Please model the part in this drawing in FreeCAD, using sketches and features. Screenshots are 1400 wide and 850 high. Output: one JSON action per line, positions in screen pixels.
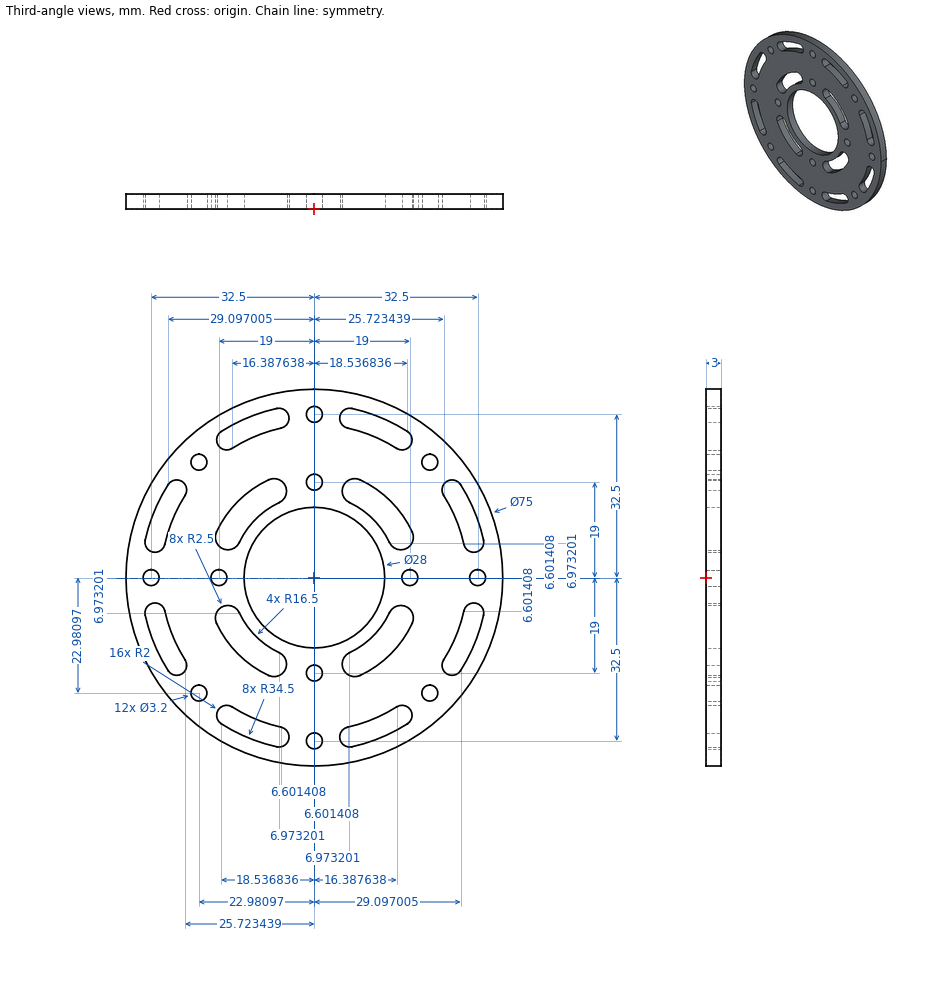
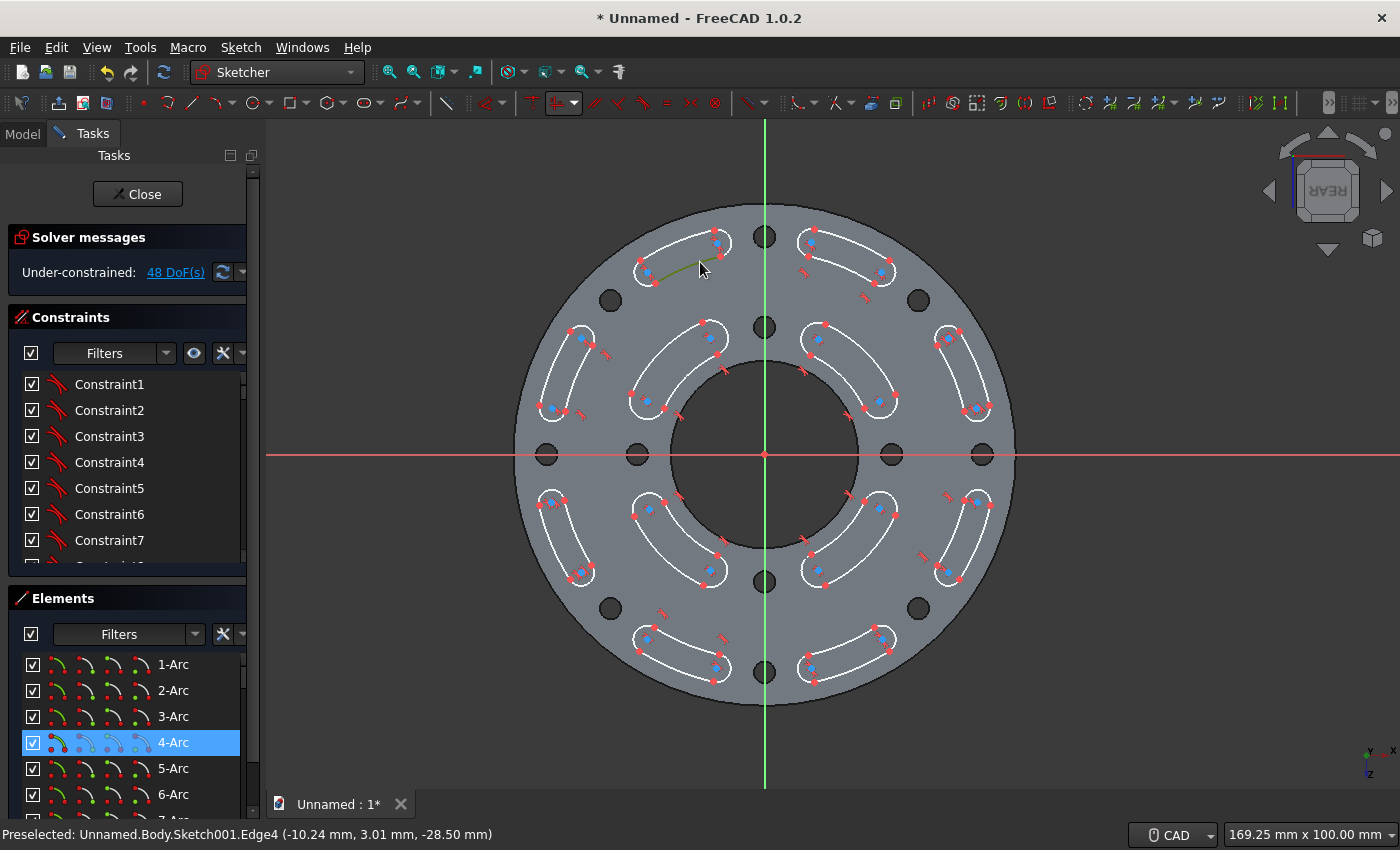
{"action": "left_click", "coordinate": [856, 273]}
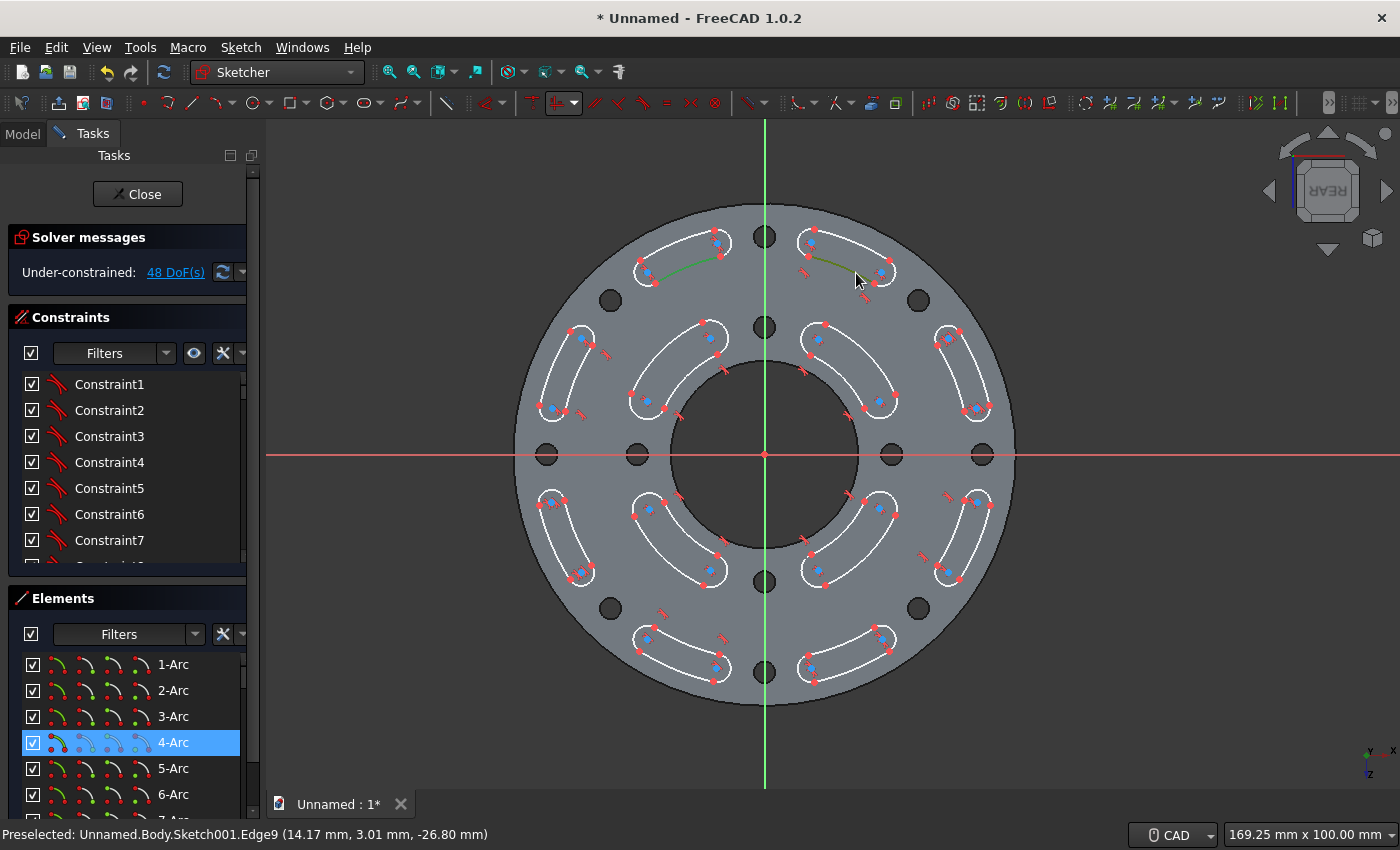
{"action": "left_click", "coordinate": [959, 391]}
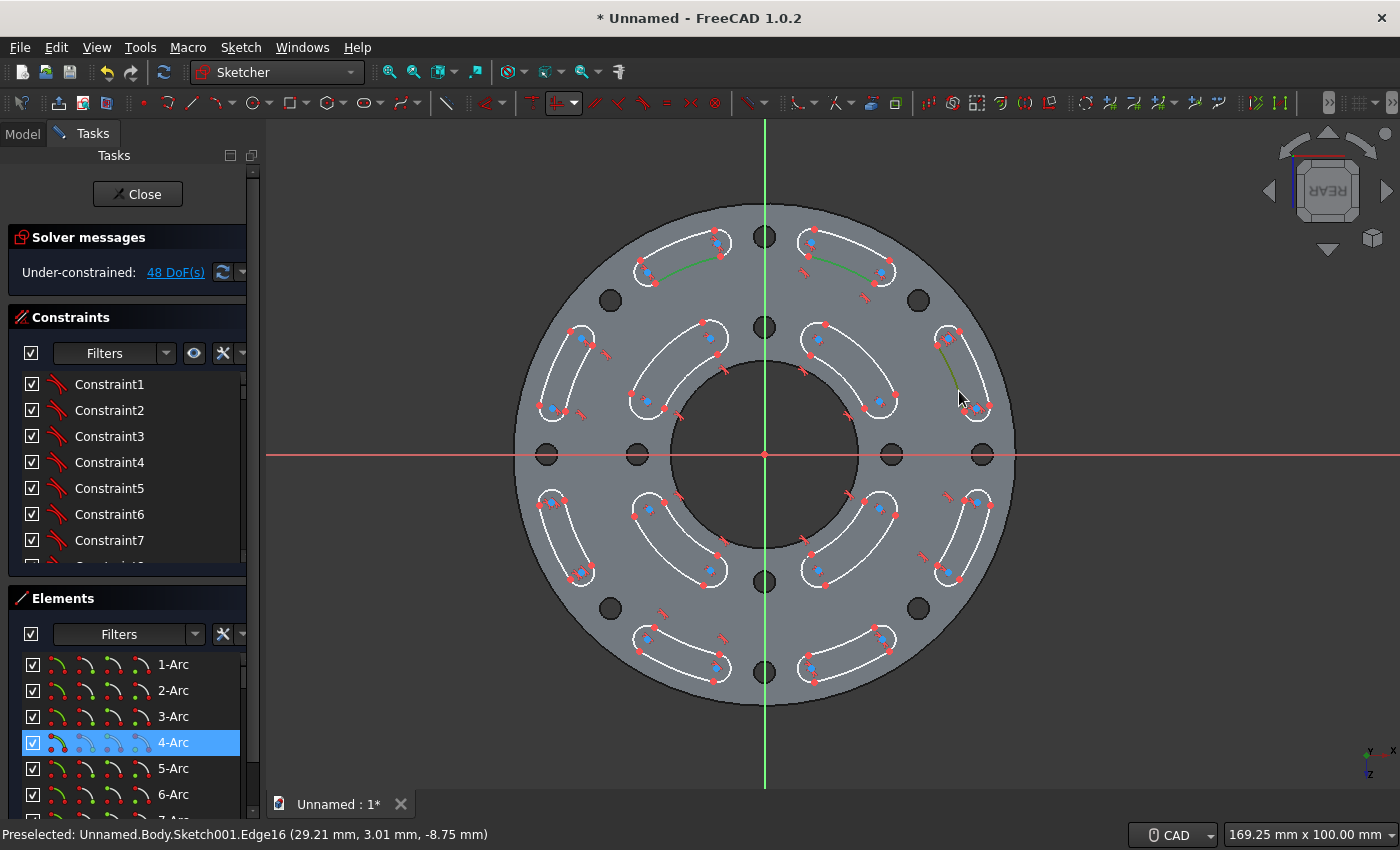
{"action": "left_click", "coordinate": [948, 547]}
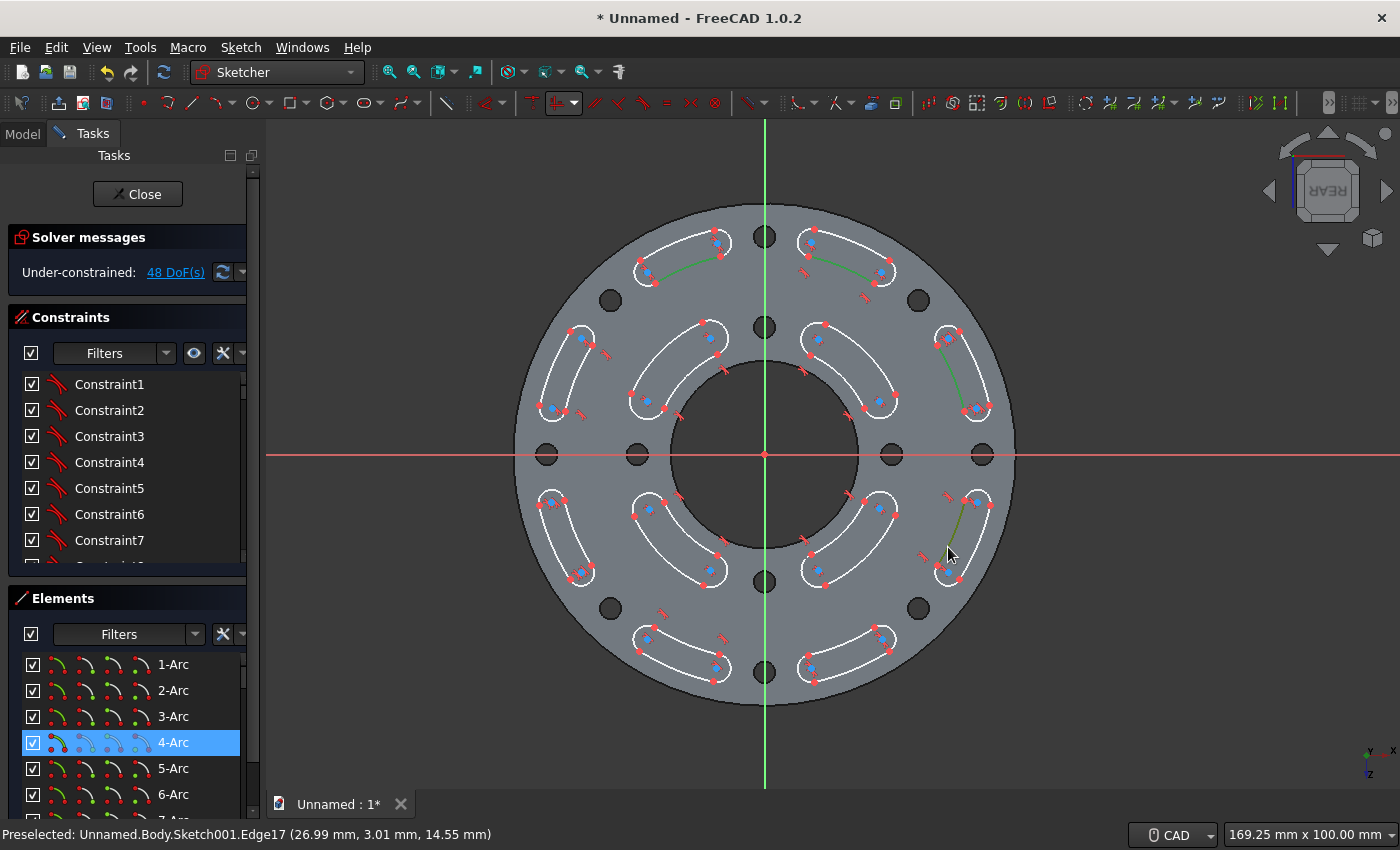
{"action": "left_click", "coordinate": [829, 649]}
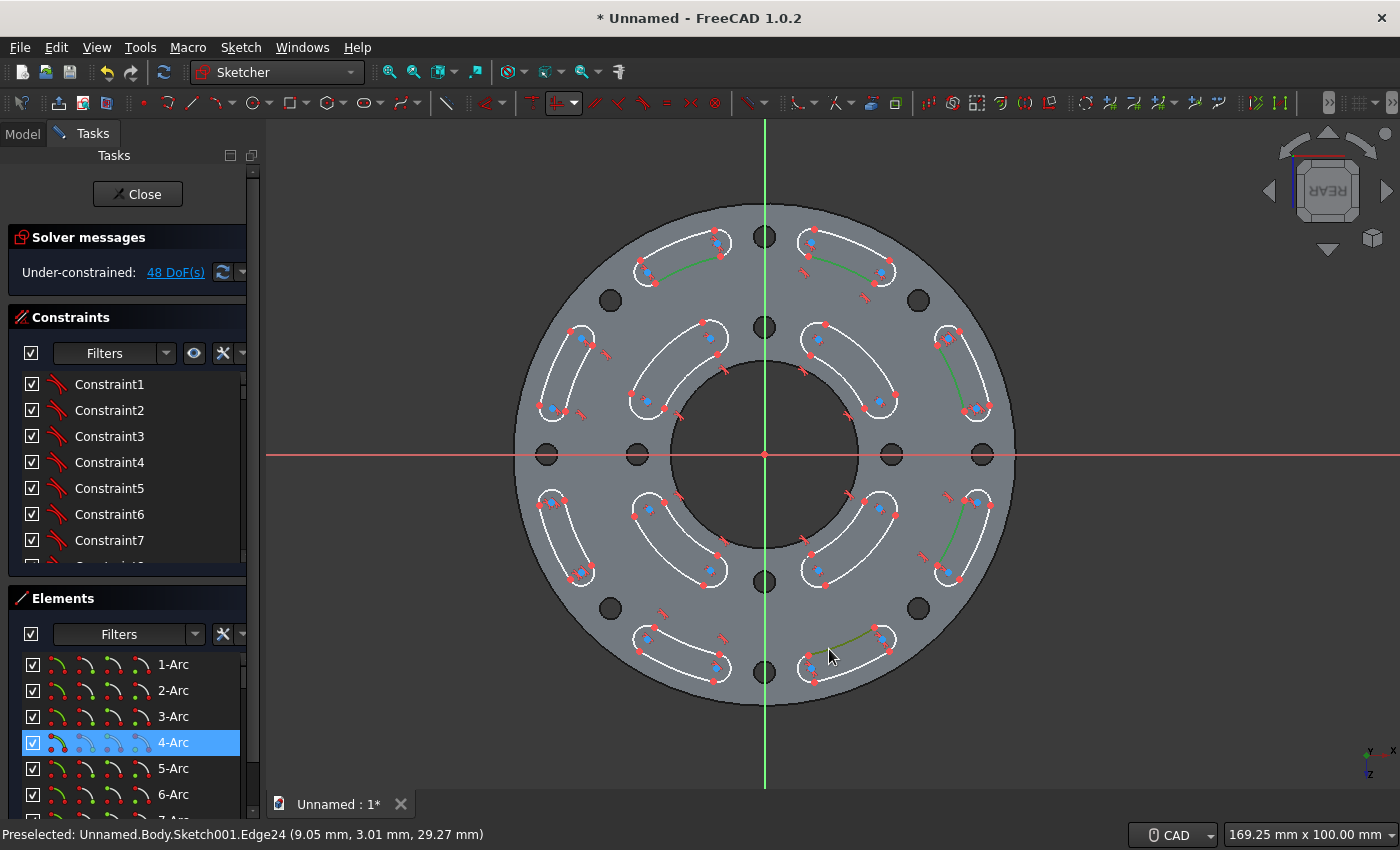
{"action": "left_click", "coordinate": [673, 638]}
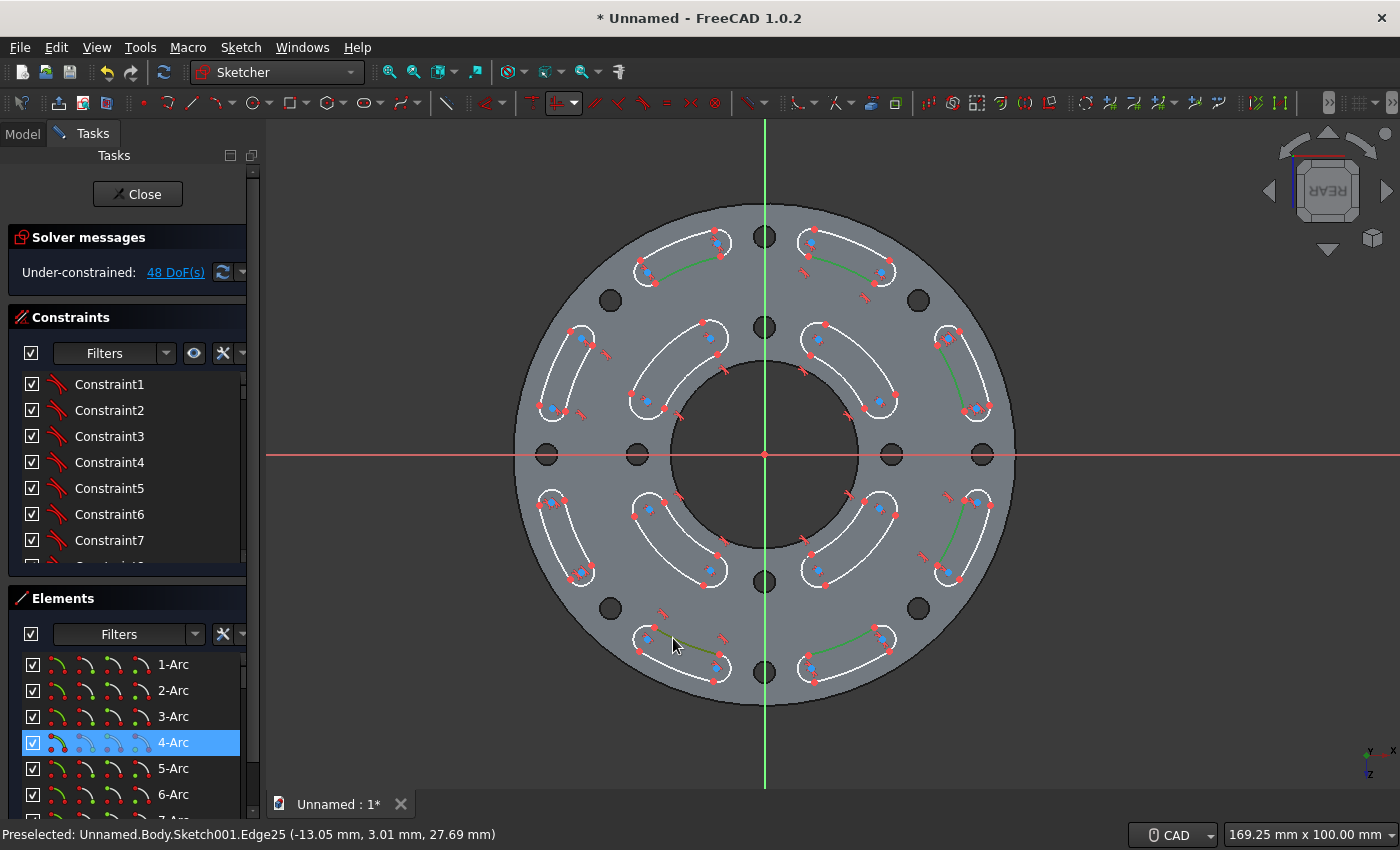
{"action": "left_click", "coordinate": [570, 521]}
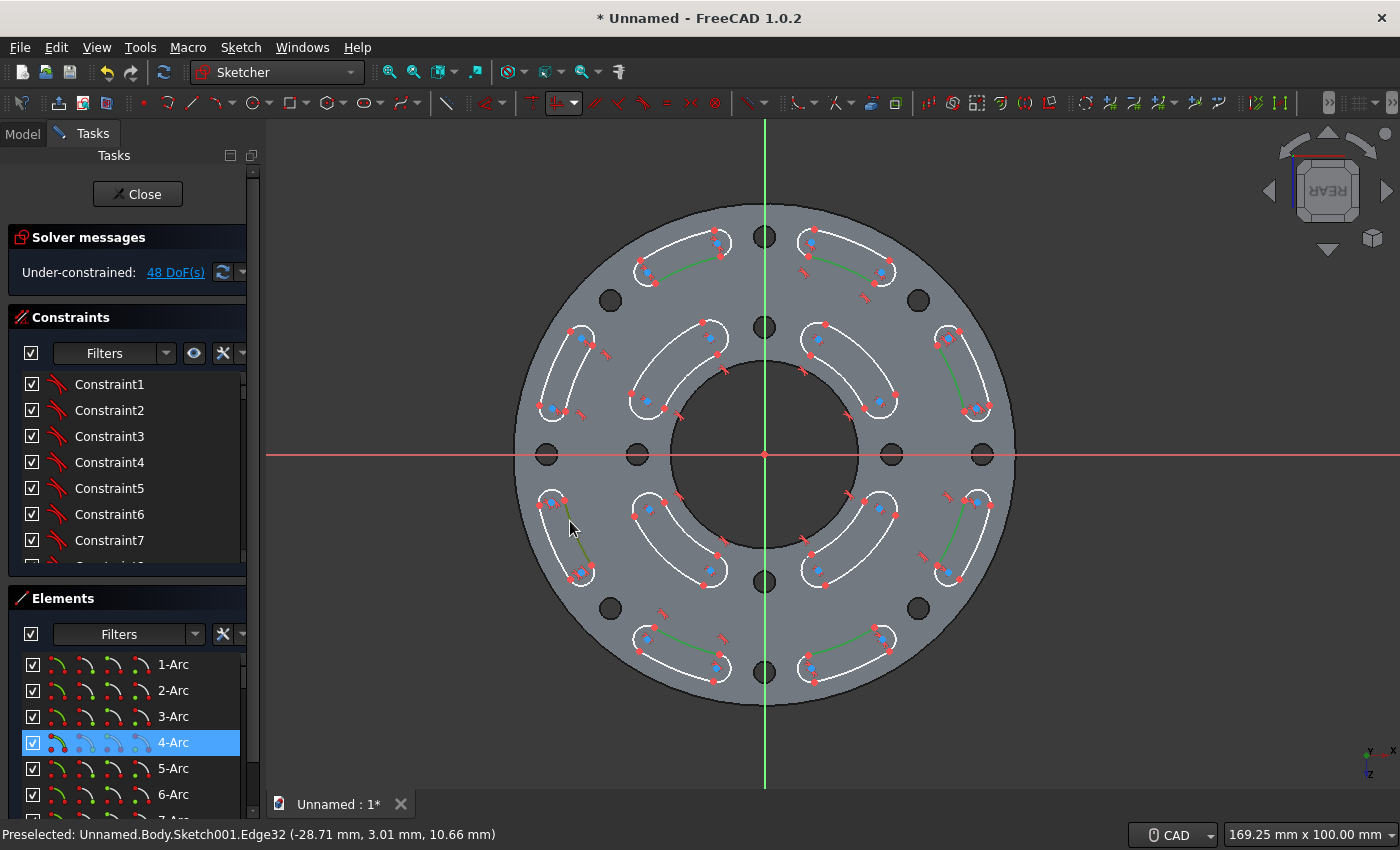
{"action": "left_click", "coordinate": [582, 364]}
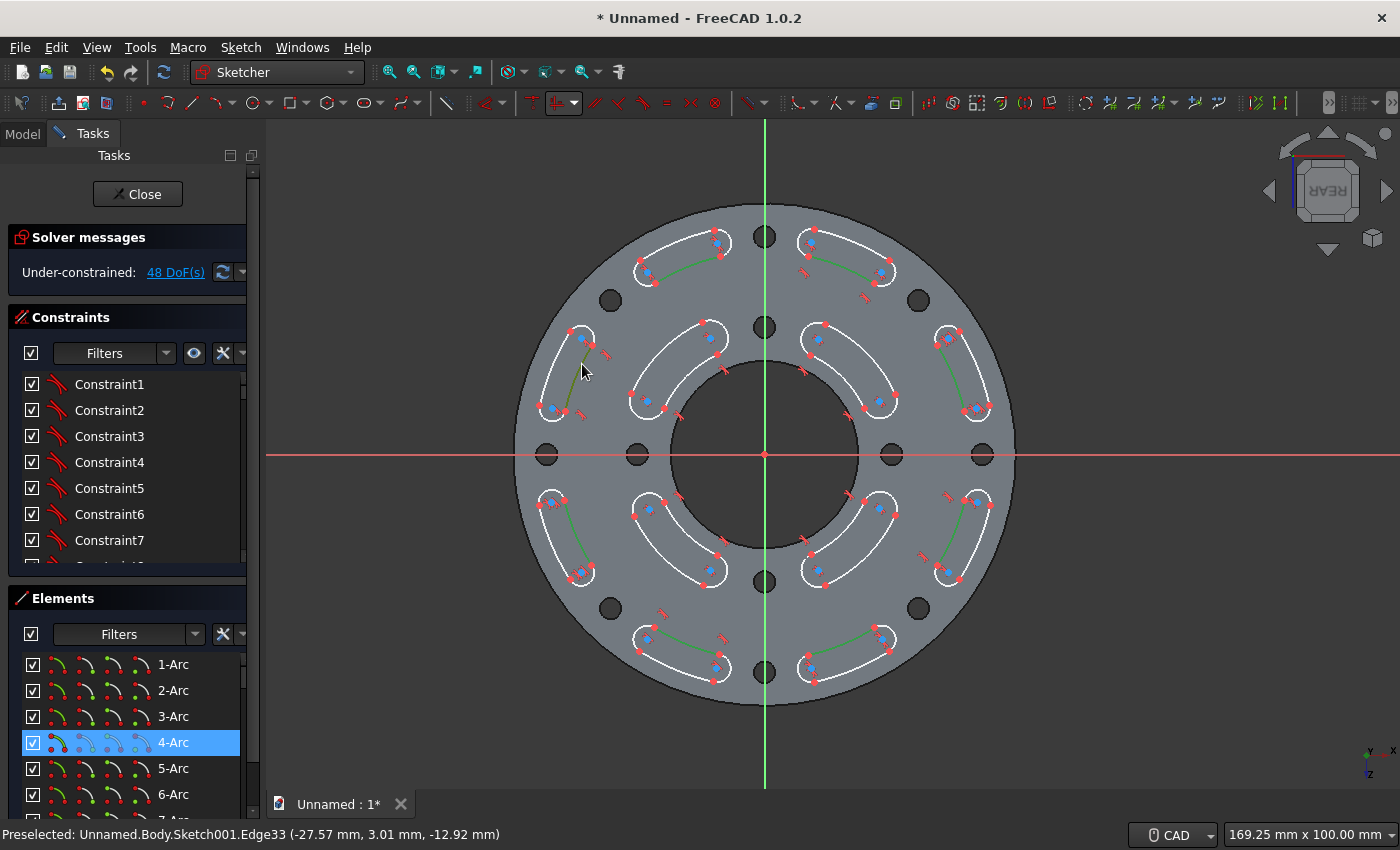
{"action": "left_click", "coordinate": [668, 104]}